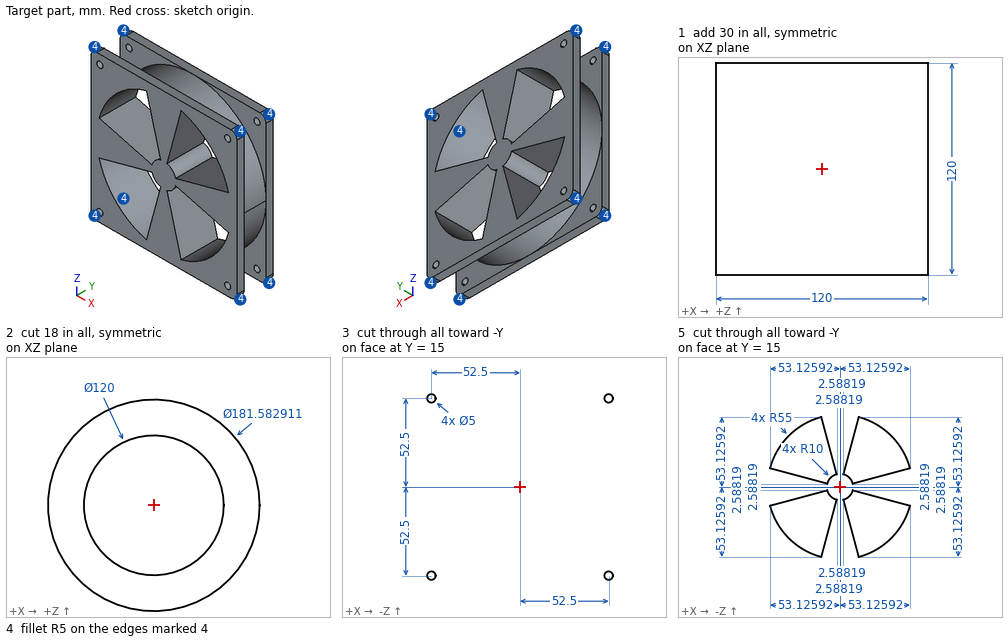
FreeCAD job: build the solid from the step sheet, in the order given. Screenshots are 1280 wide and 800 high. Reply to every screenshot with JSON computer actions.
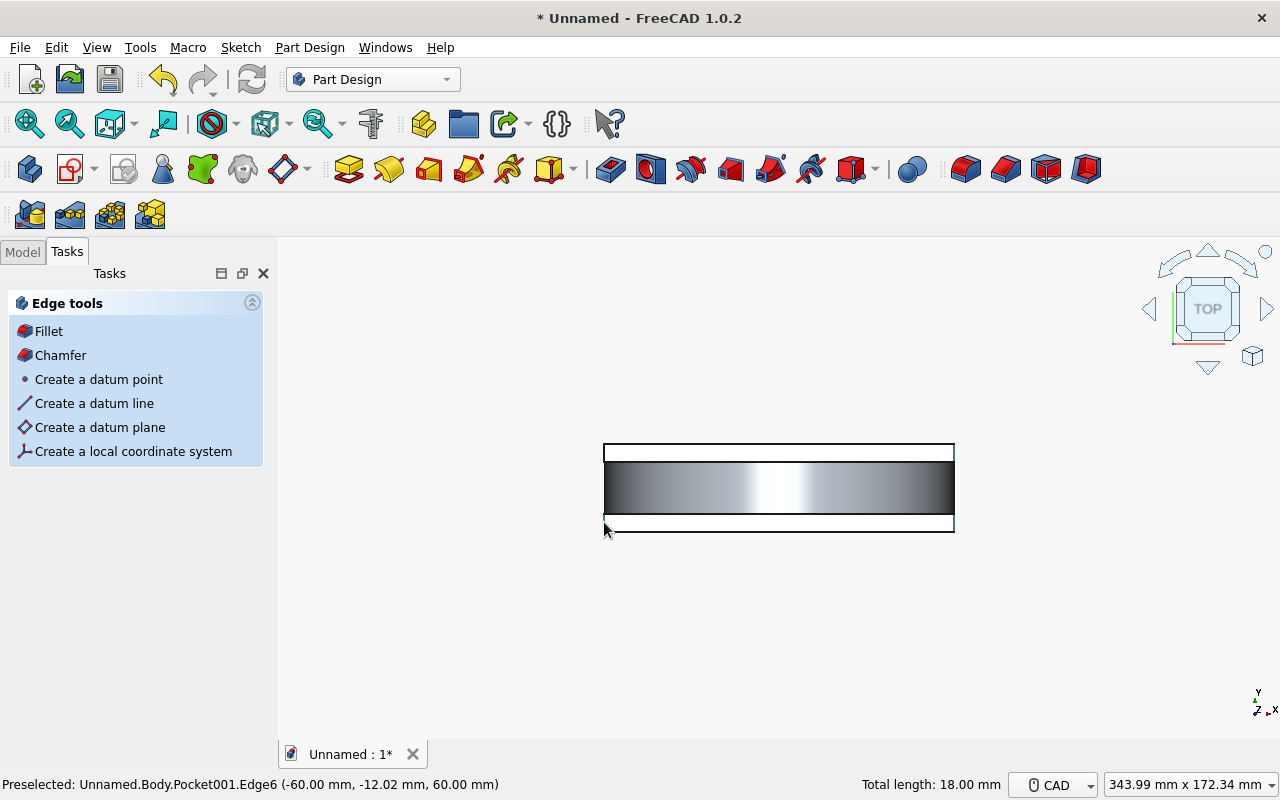
{"action": "left_click", "coordinate": [604, 452], "text": "ctrl"}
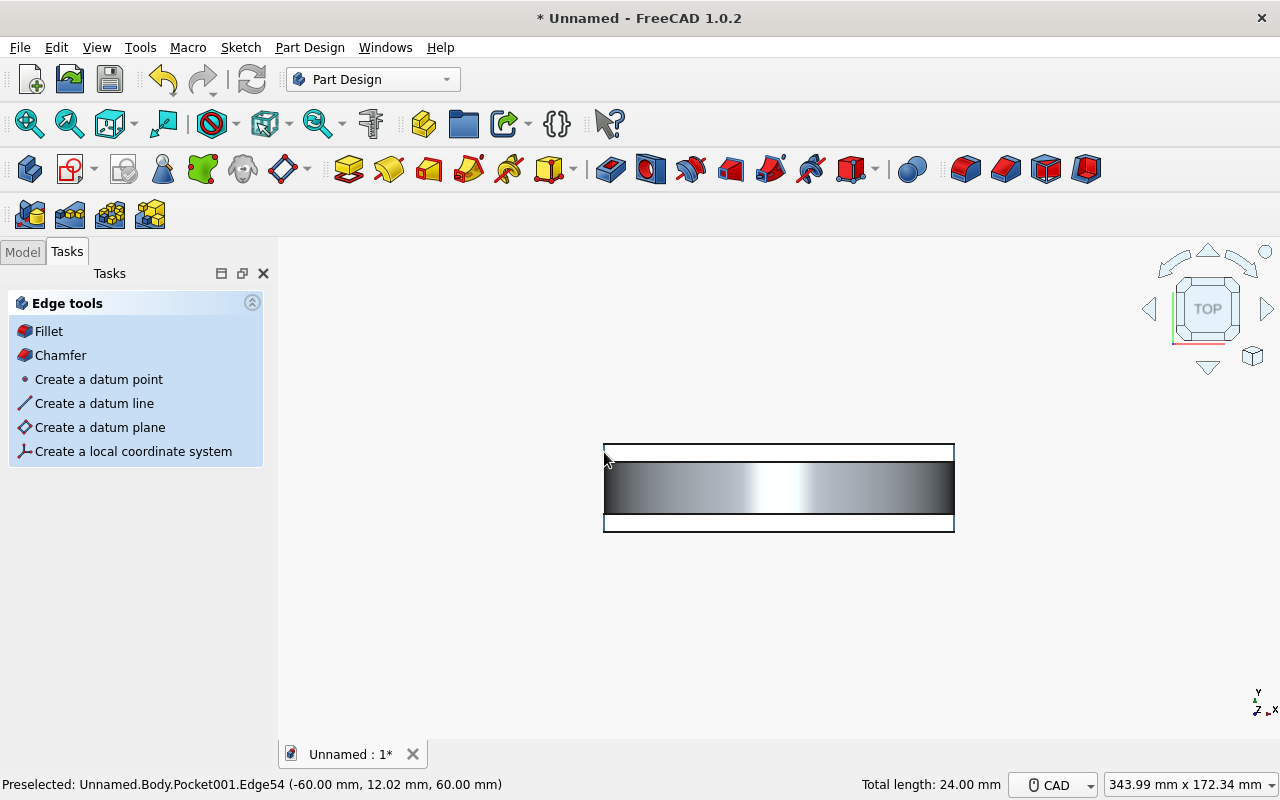
{"action": "scroll", "coordinate": [604, 522], "scroll_direction": "up", "scroll_amount": 5}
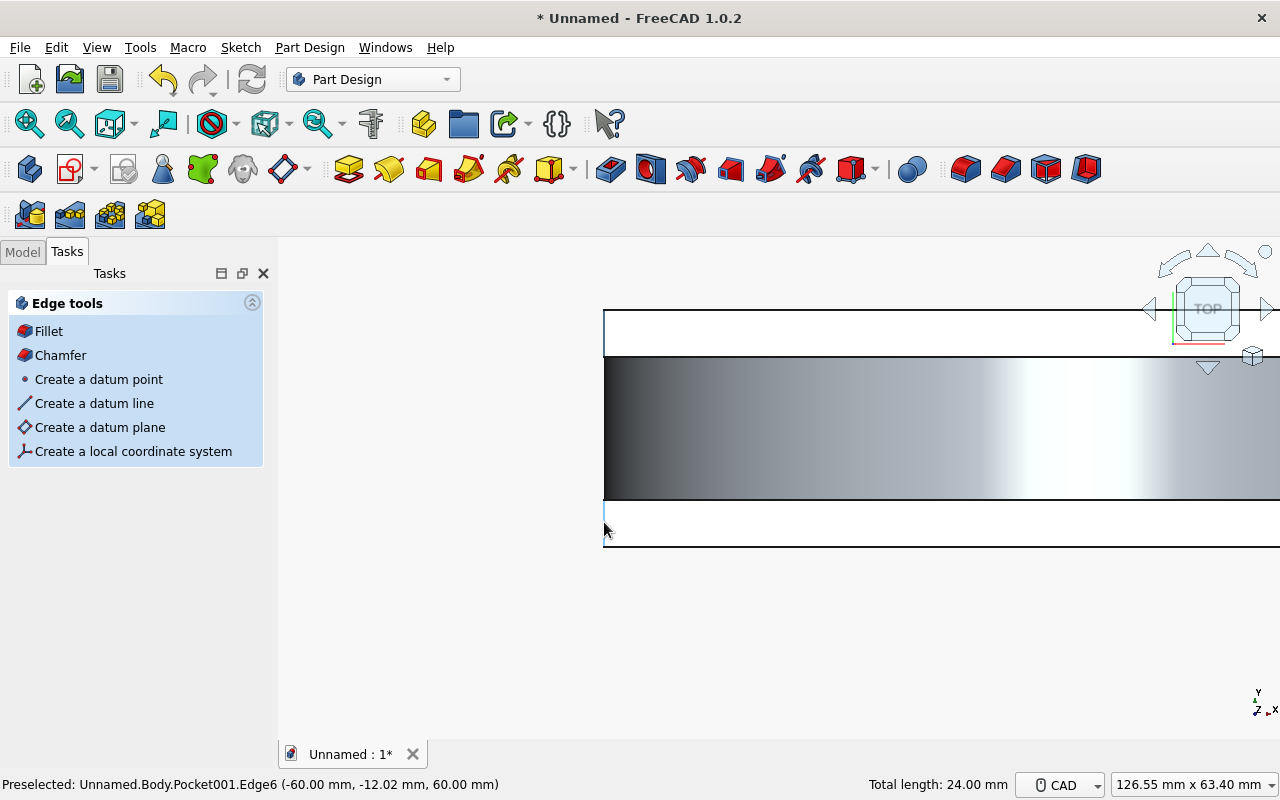
{"action": "left_click", "coordinate": [30, 124]}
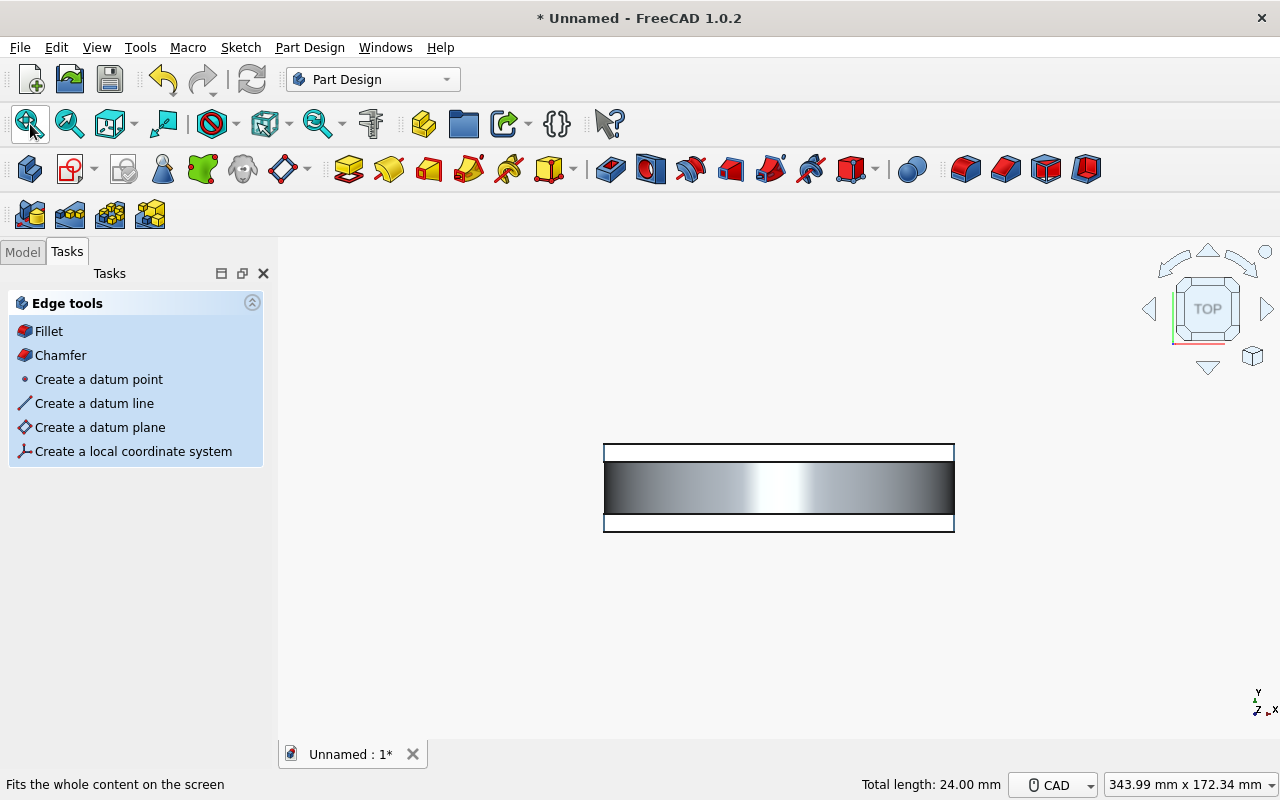
{"action": "key", "text": "1"}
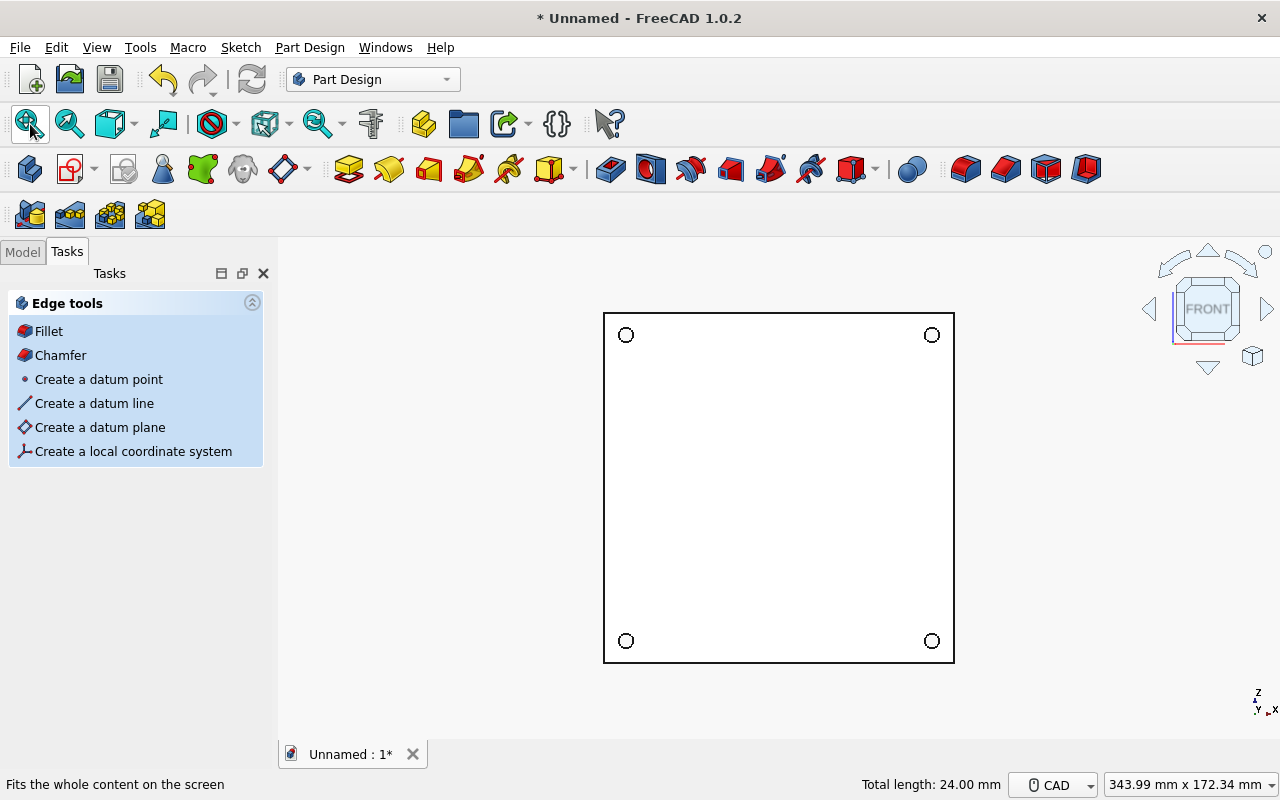
{"action": "scroll", "coordinate": [604, 662], "scroll_direction": "up", "scroll_amount": 5}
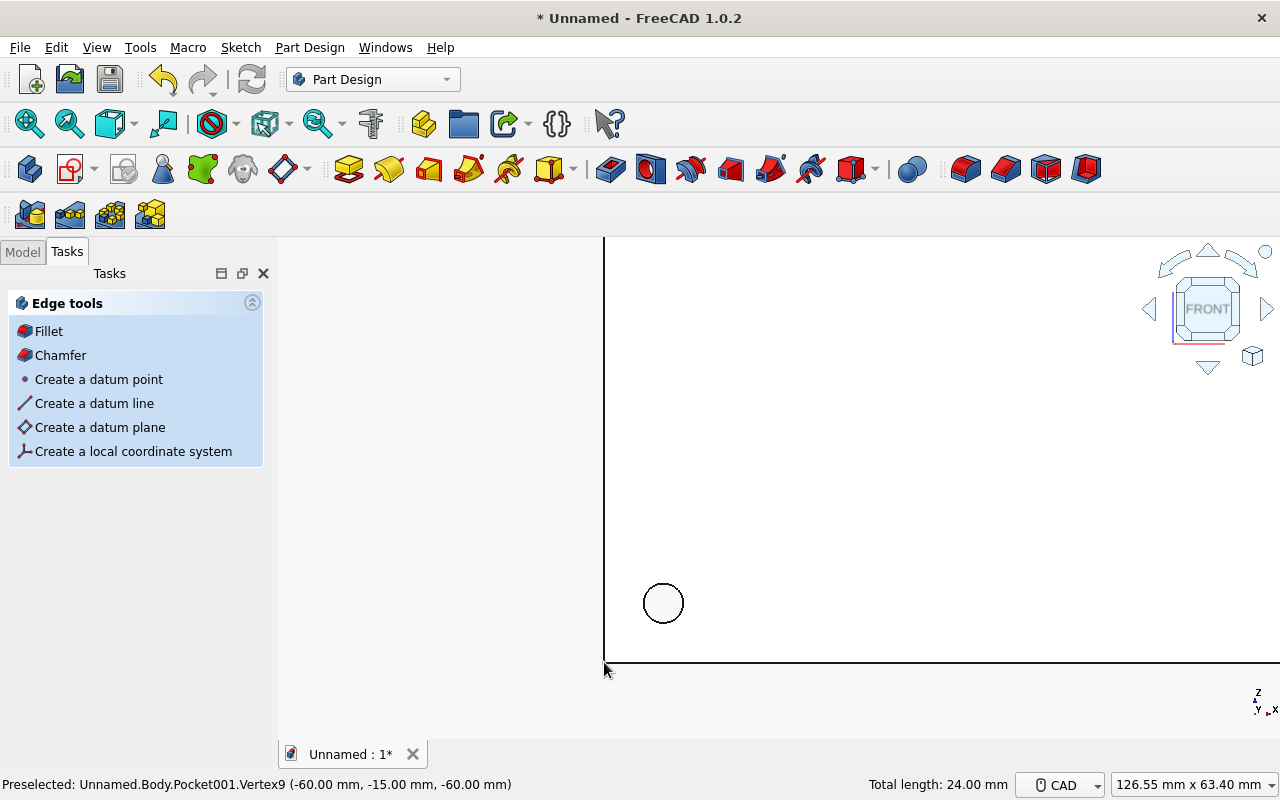
{"action": "left_click", "coordinate": [30, 124]}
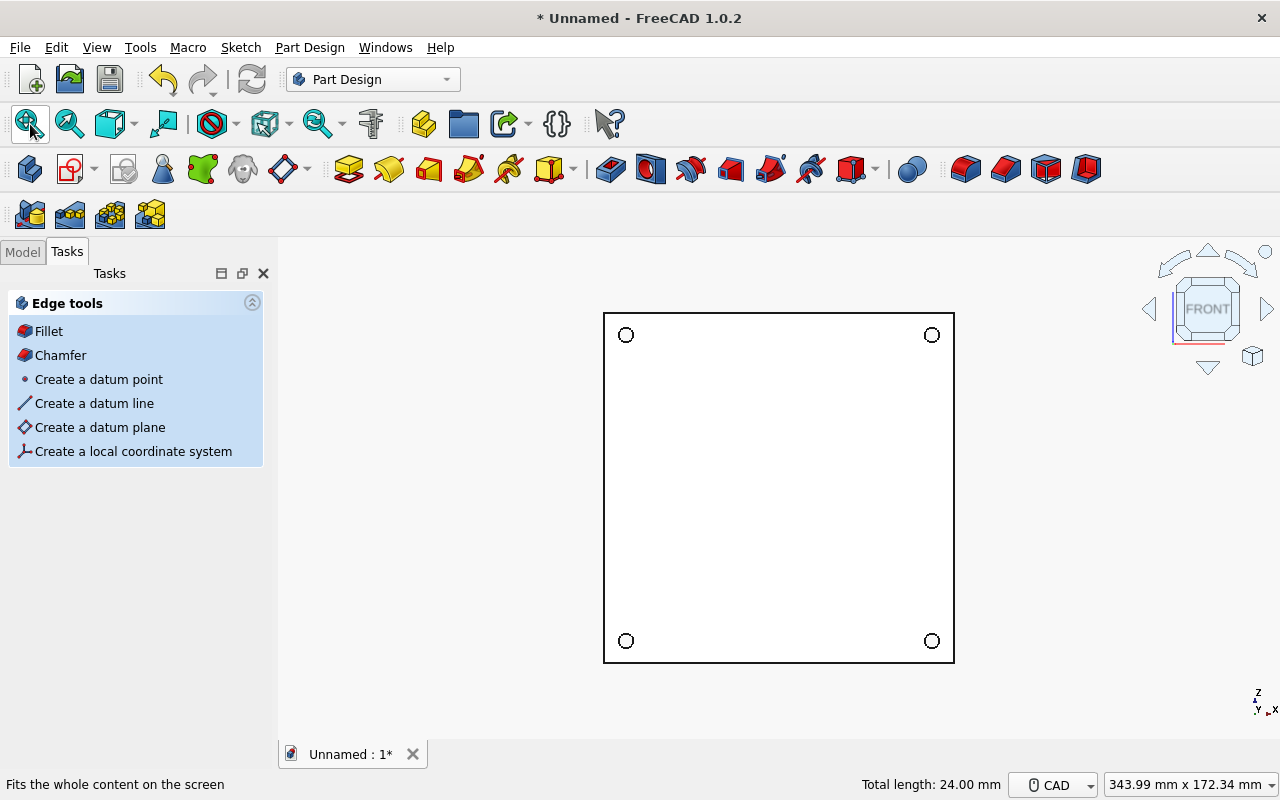
{"action": "key", "text": "3"}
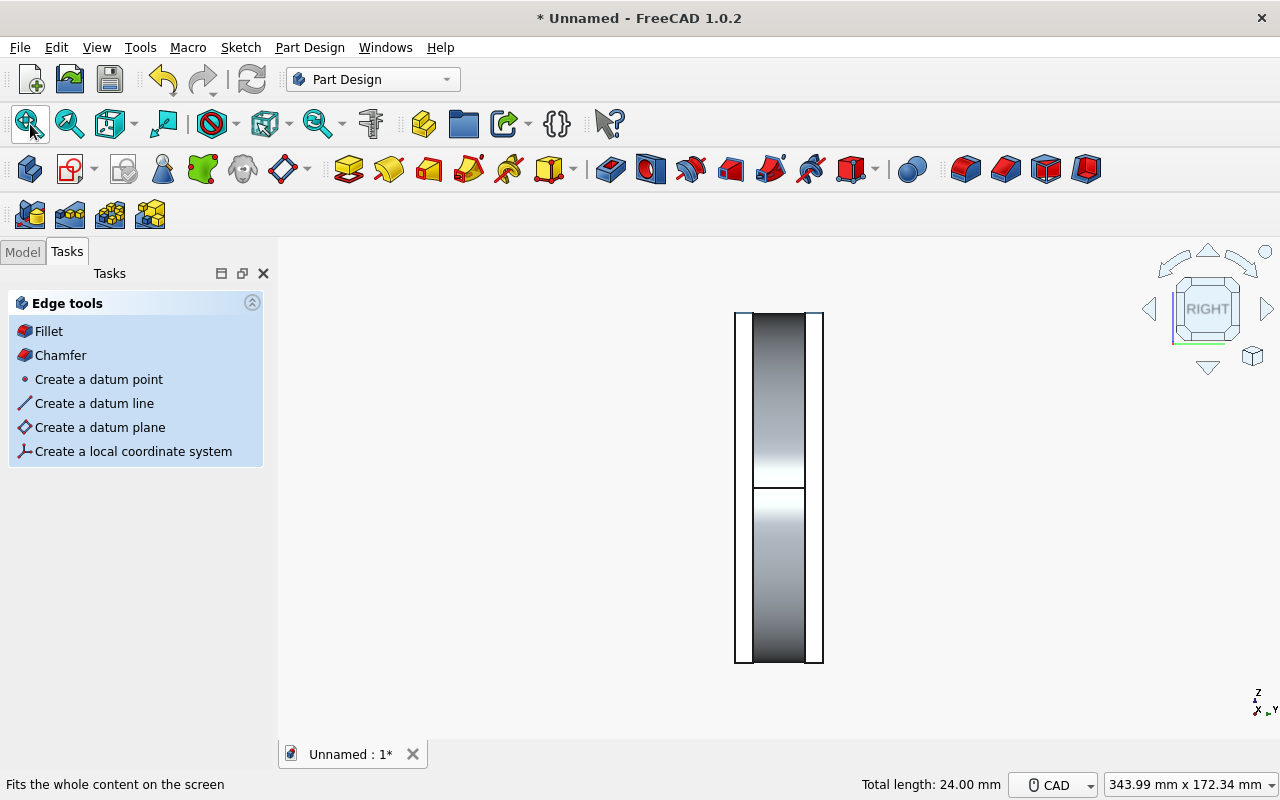
{"action": "left_click", "coordinate": [744, 662], "text": "ctrl"}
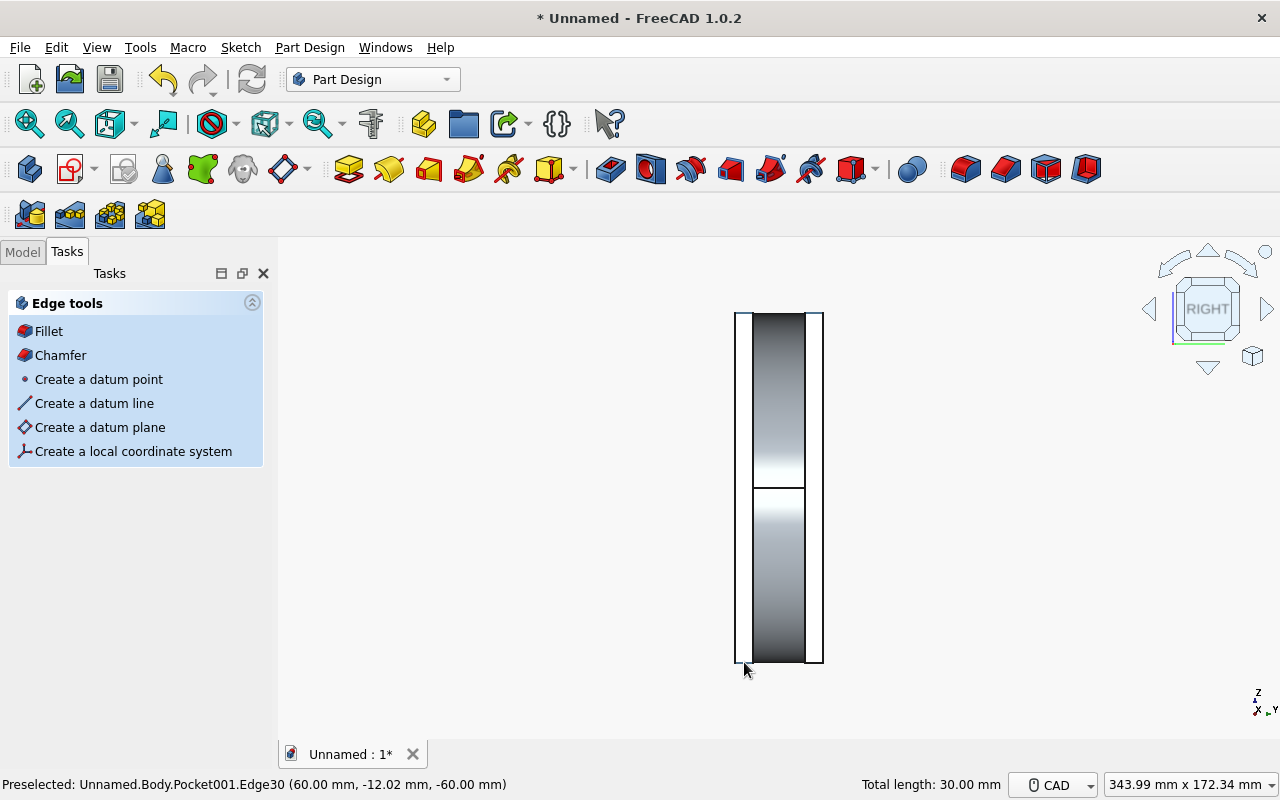
{"action": "left_click", "coordinate": [814, 662], "text": "ctrl"}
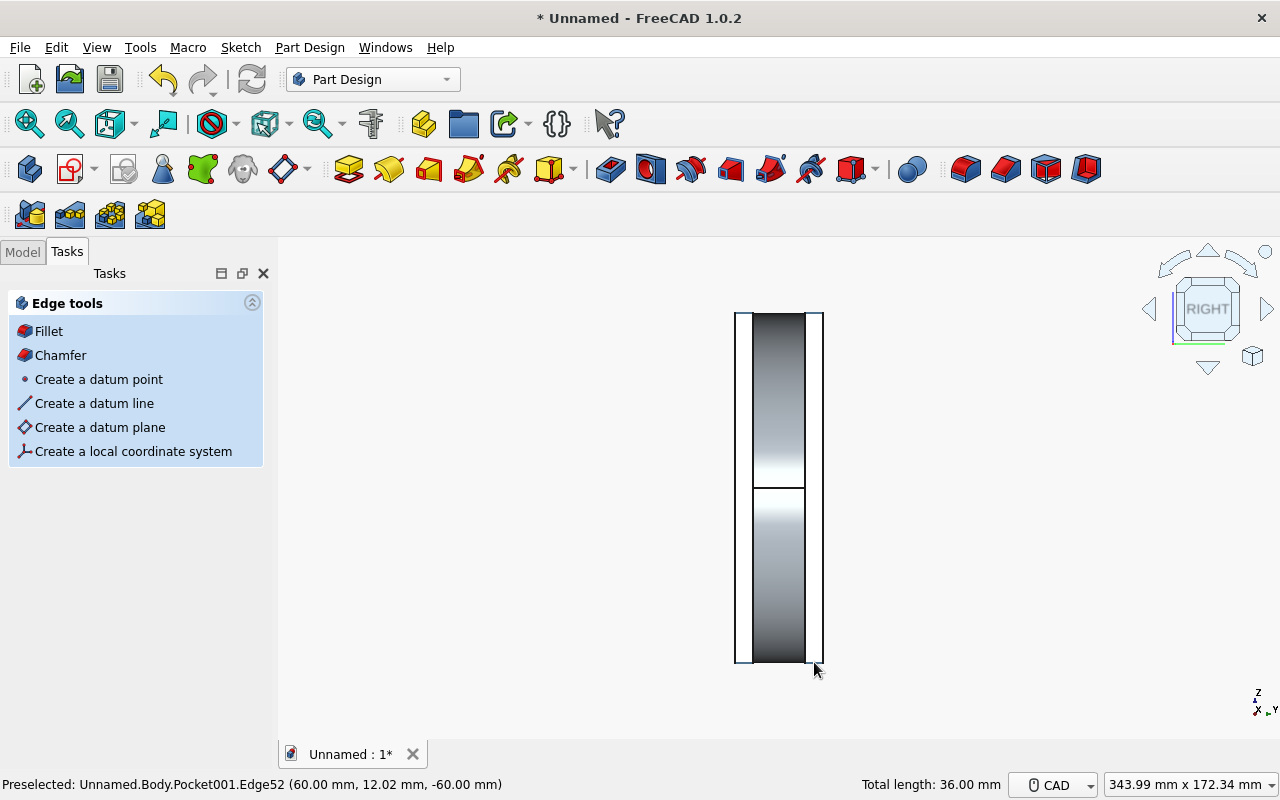
{"action": "scroll", "coordinate": [744, 662], "scroll_direction": "up", "scroll_amount": 5}